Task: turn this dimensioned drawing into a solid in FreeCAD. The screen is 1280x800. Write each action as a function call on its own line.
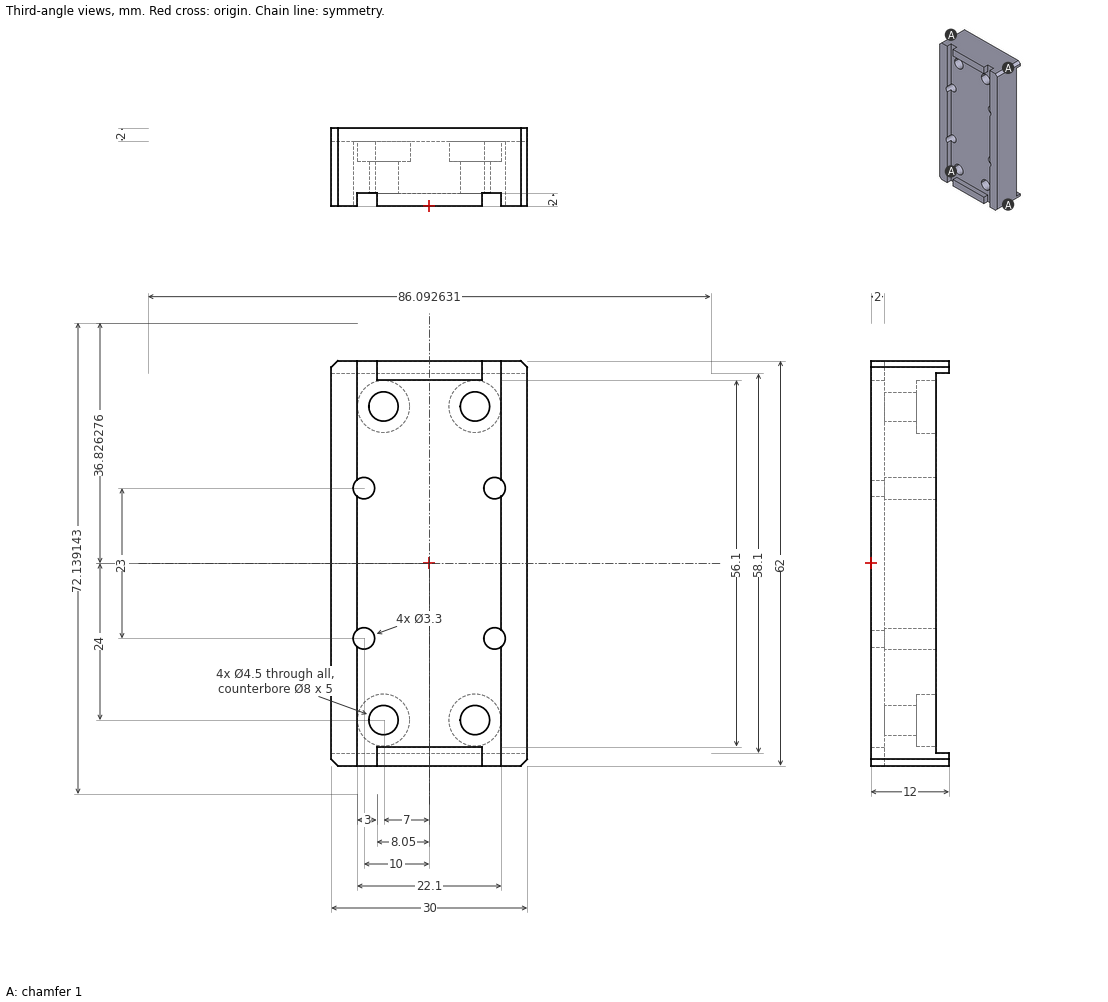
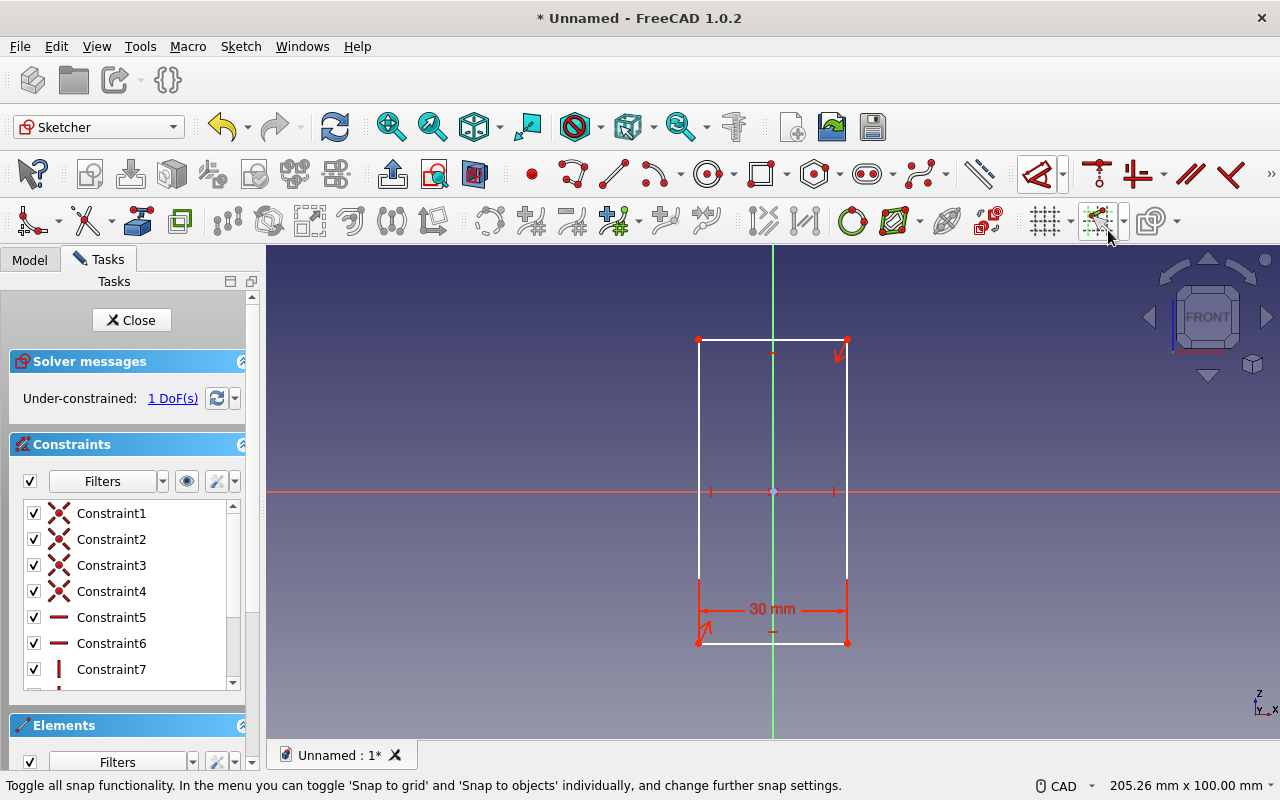
click(847, 553)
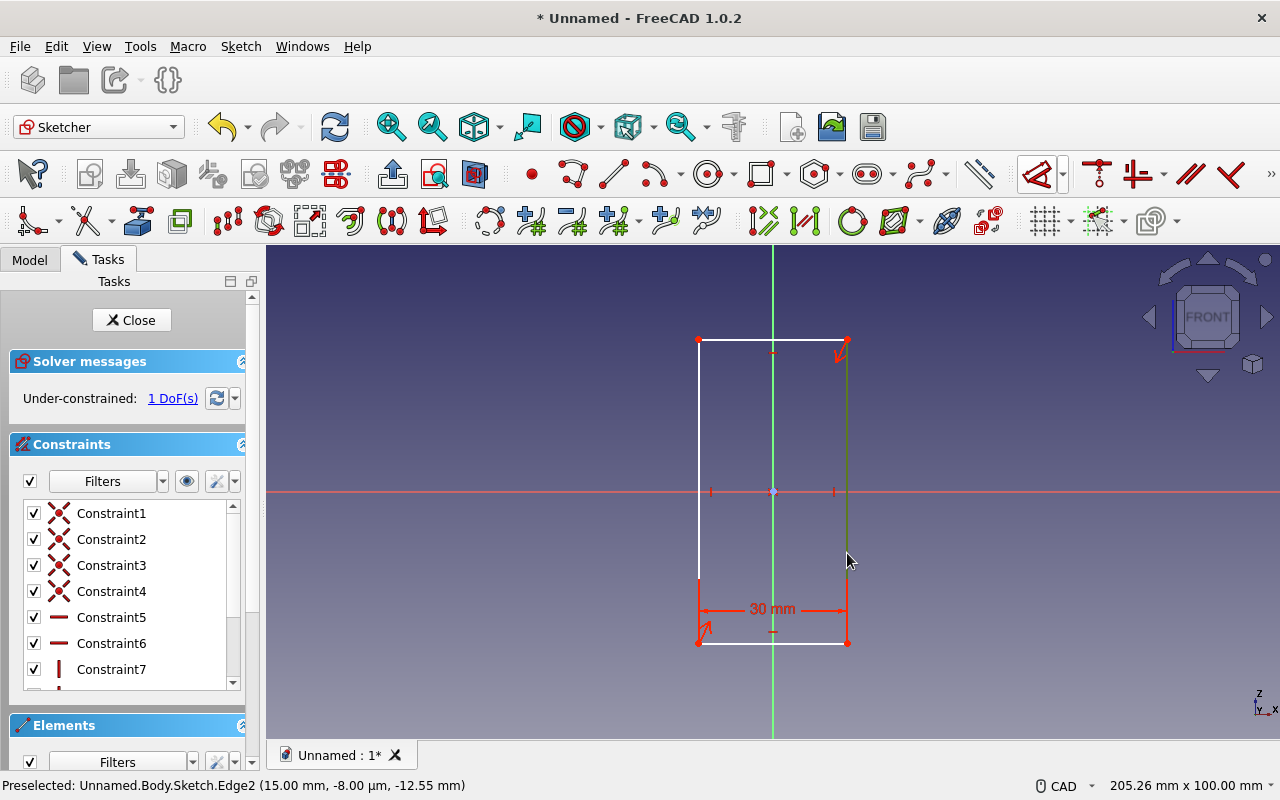
key(i)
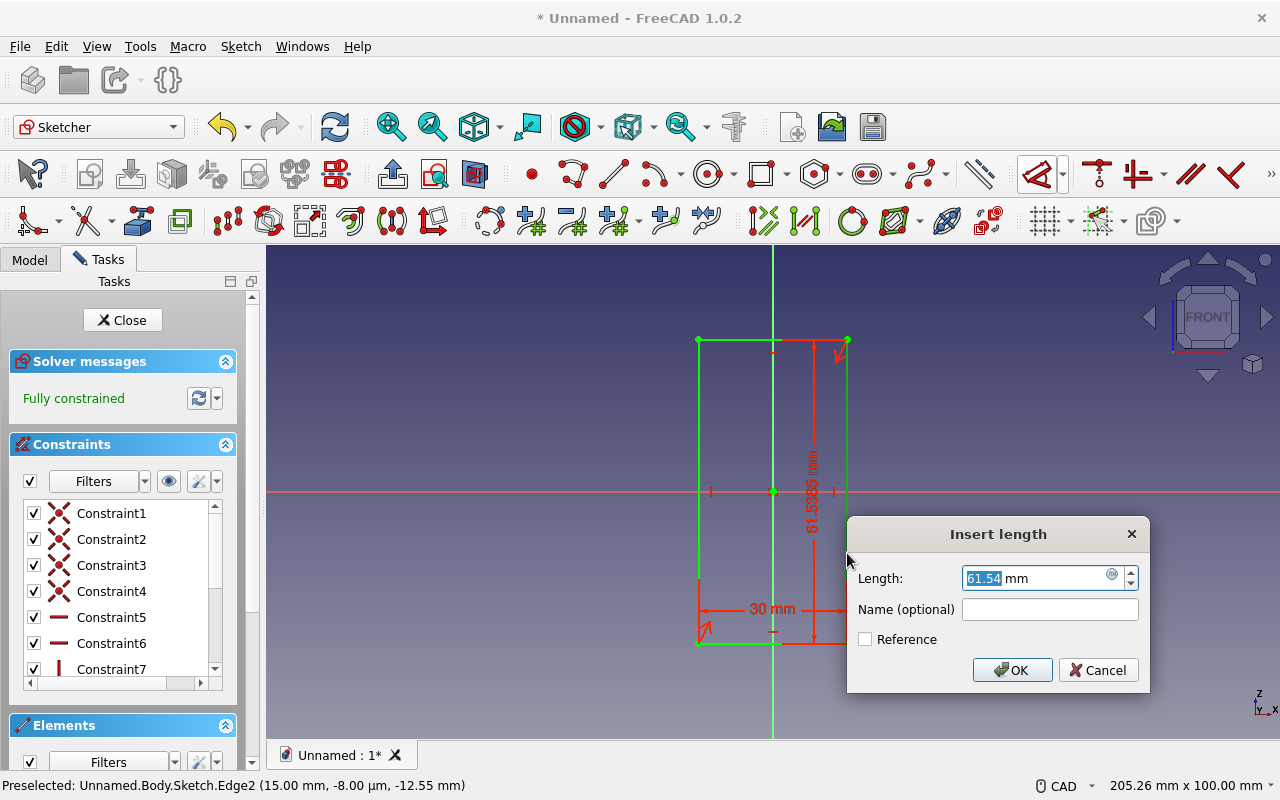
text(62)
key(Return)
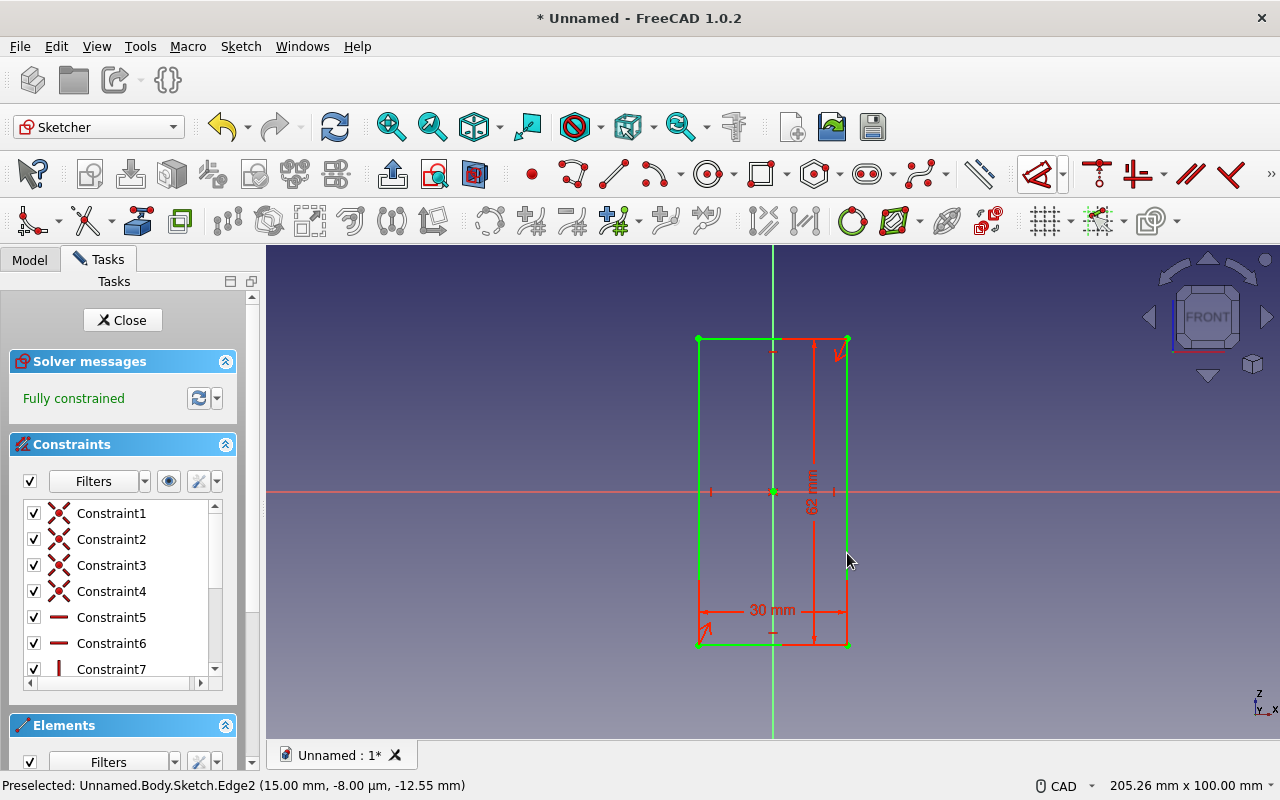
click(123, 320)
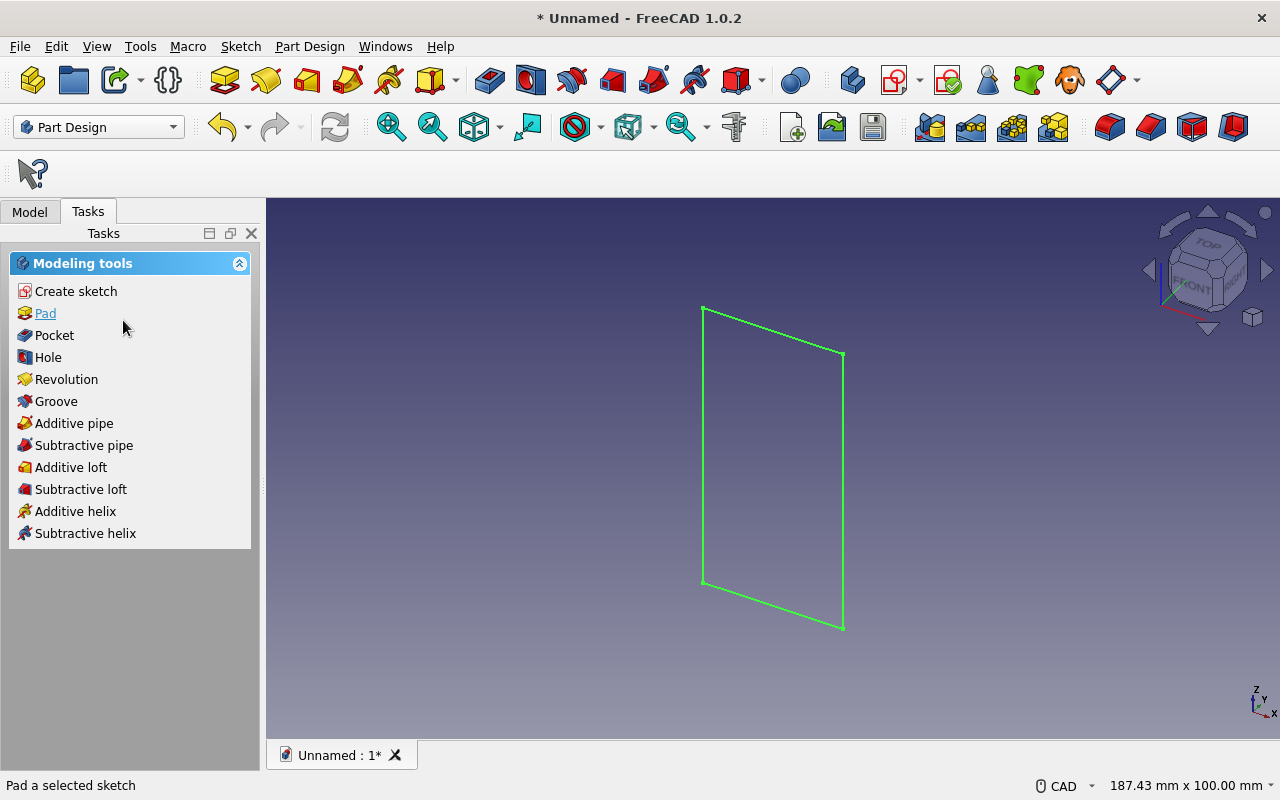
click(225, 80)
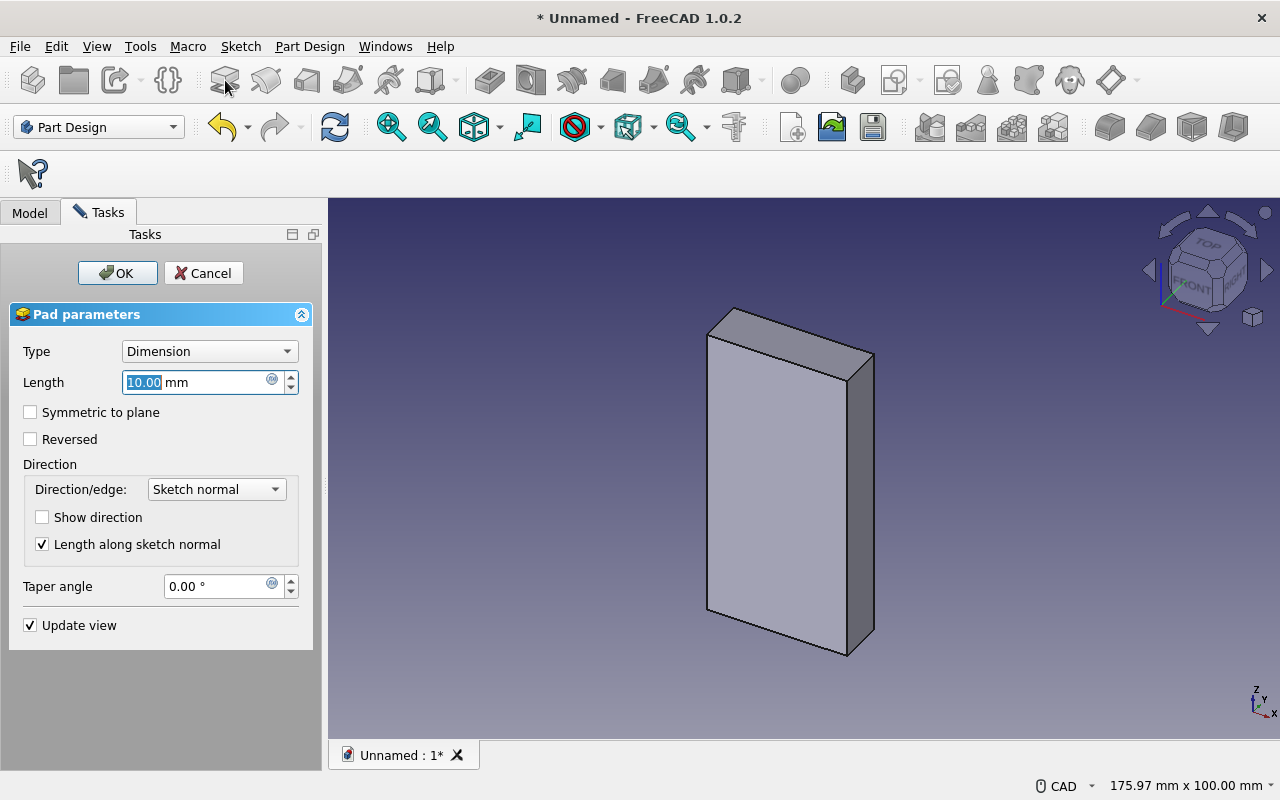
text(12)
key(Tab)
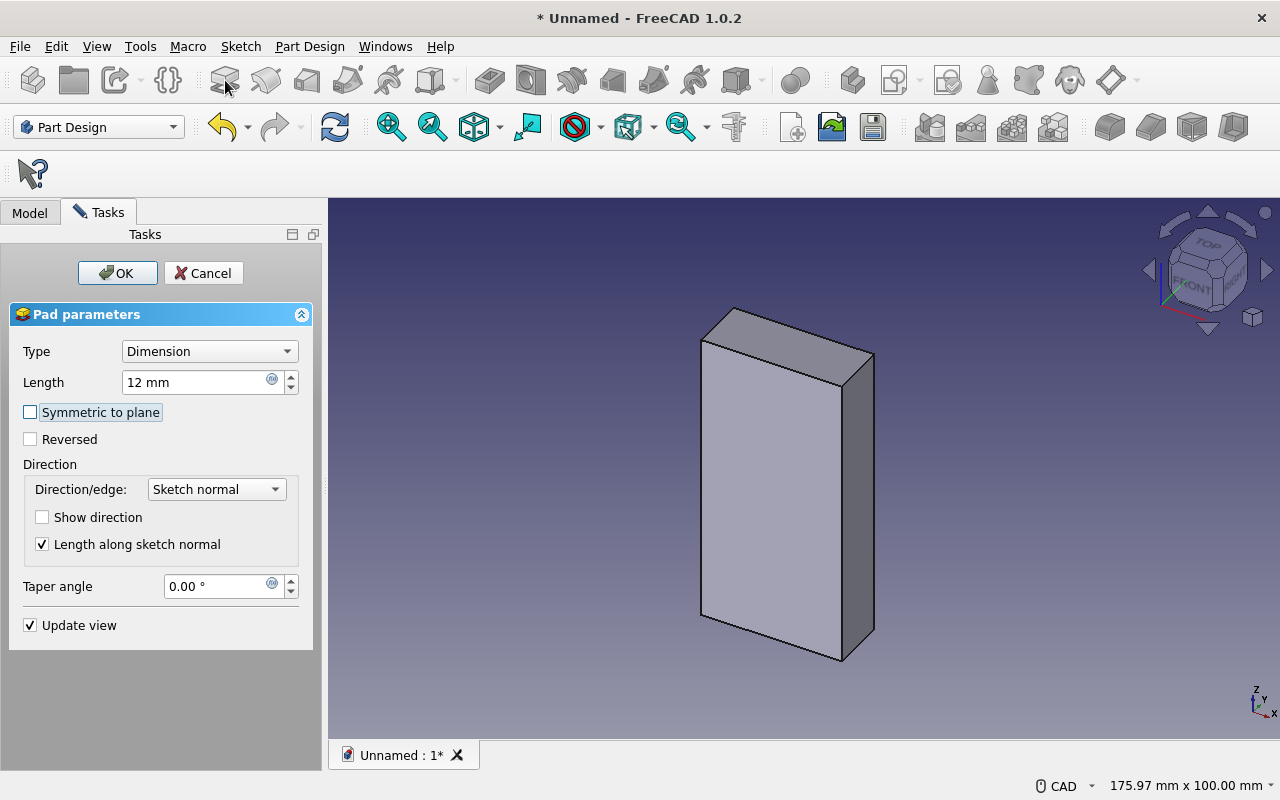
click(31, 439)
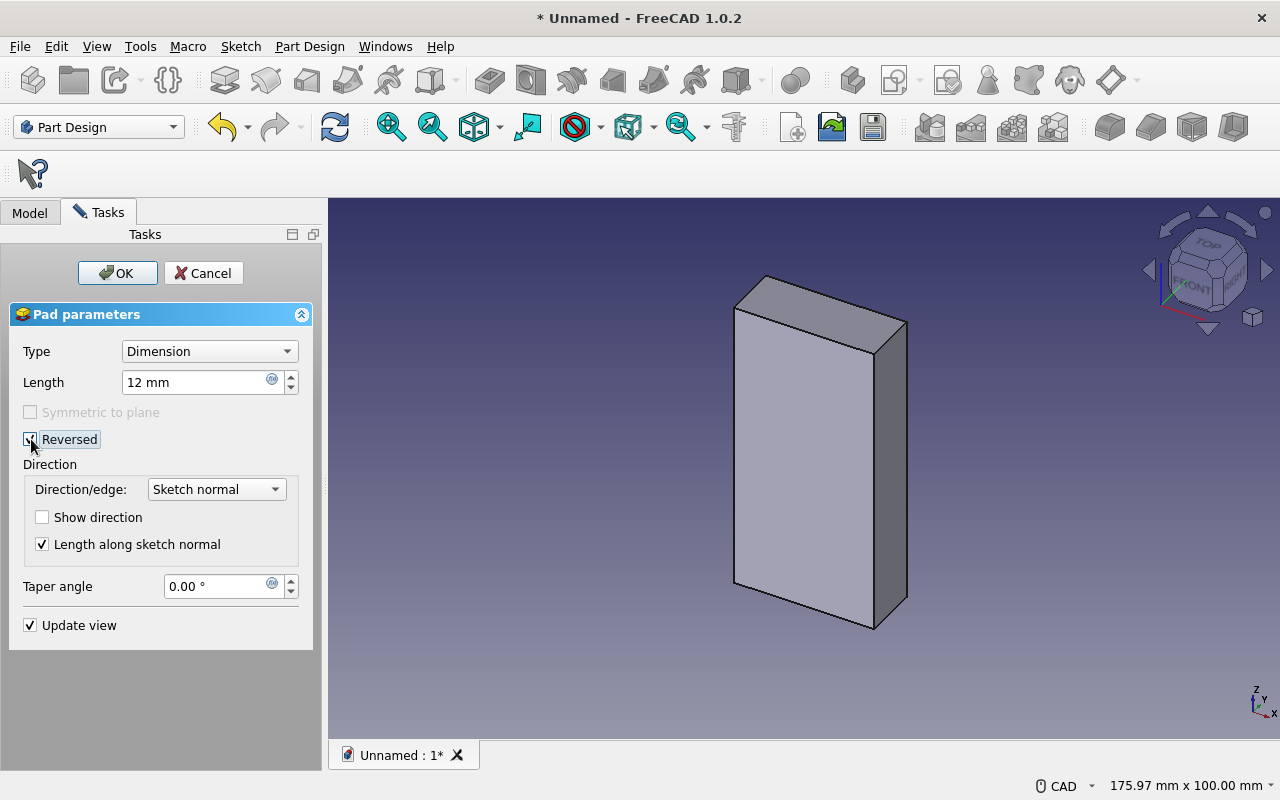
click(118, 273)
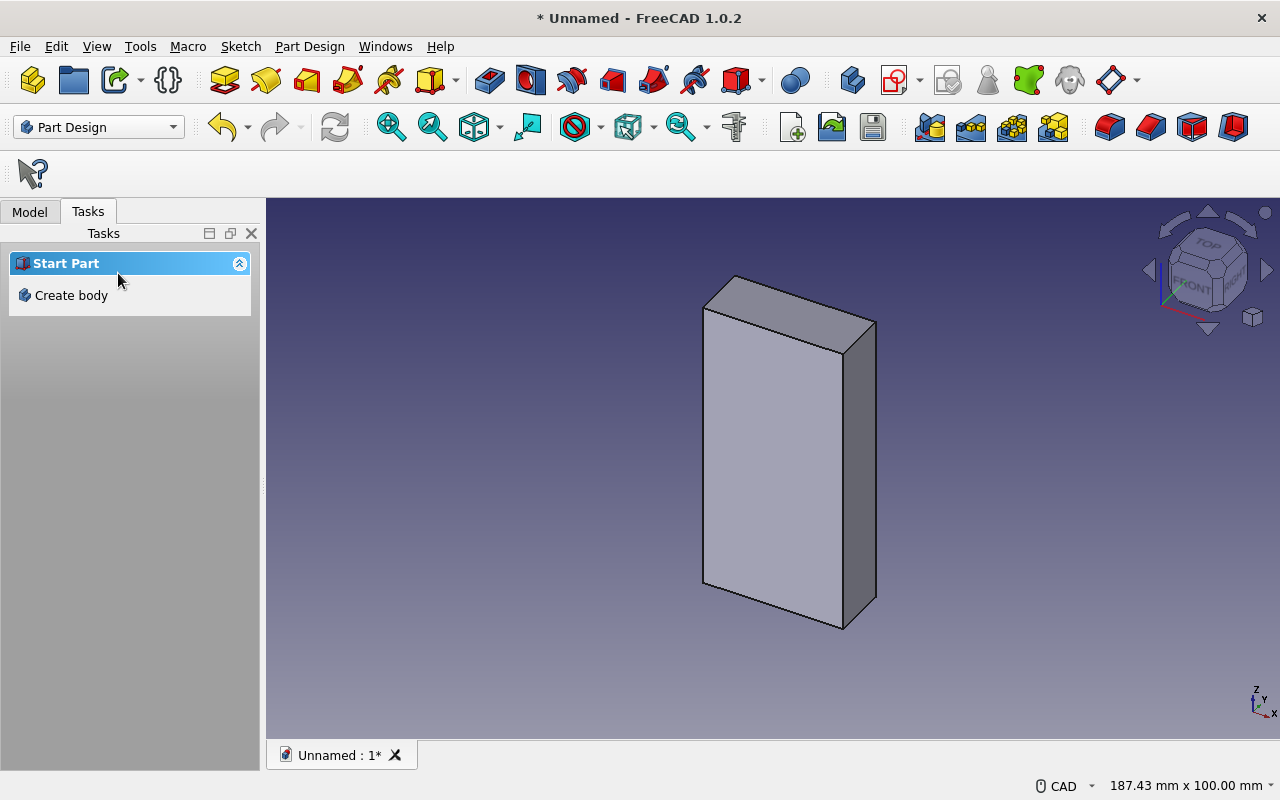
click(894, 80)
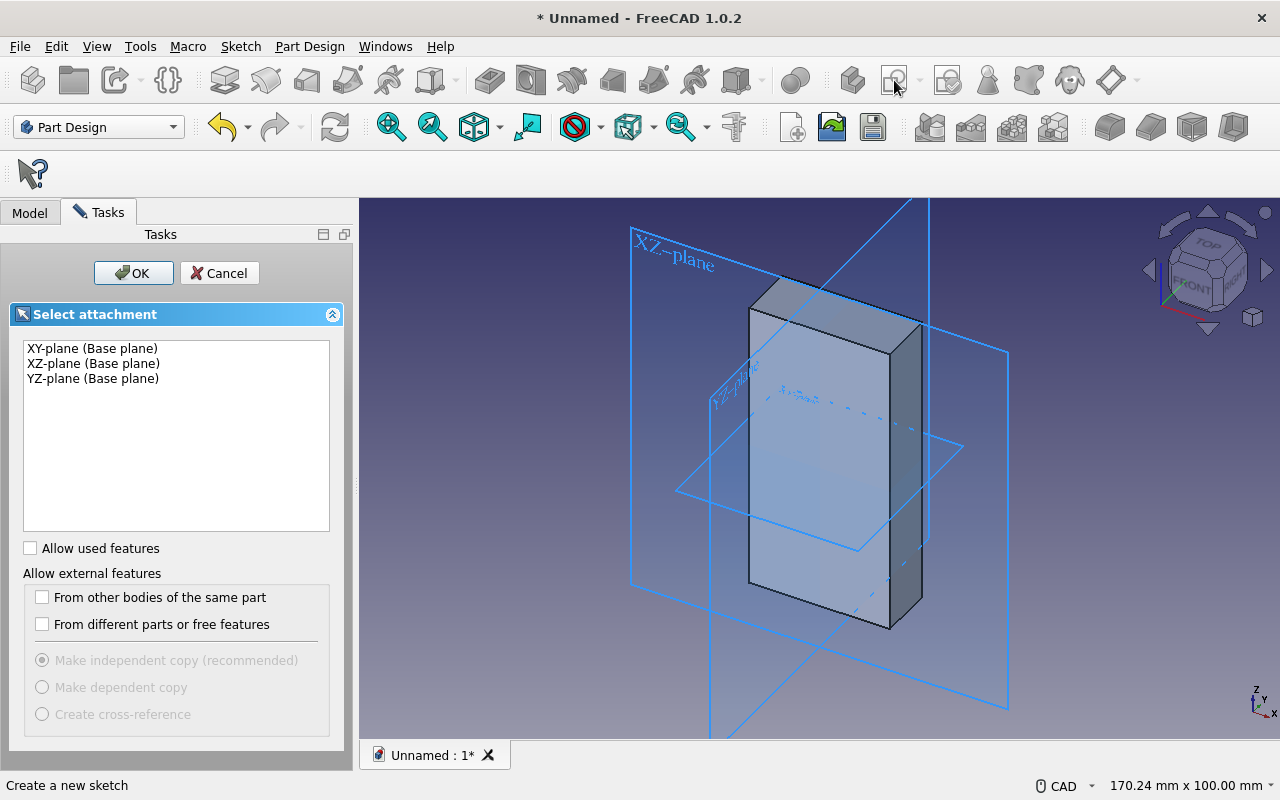
click(84, 364)